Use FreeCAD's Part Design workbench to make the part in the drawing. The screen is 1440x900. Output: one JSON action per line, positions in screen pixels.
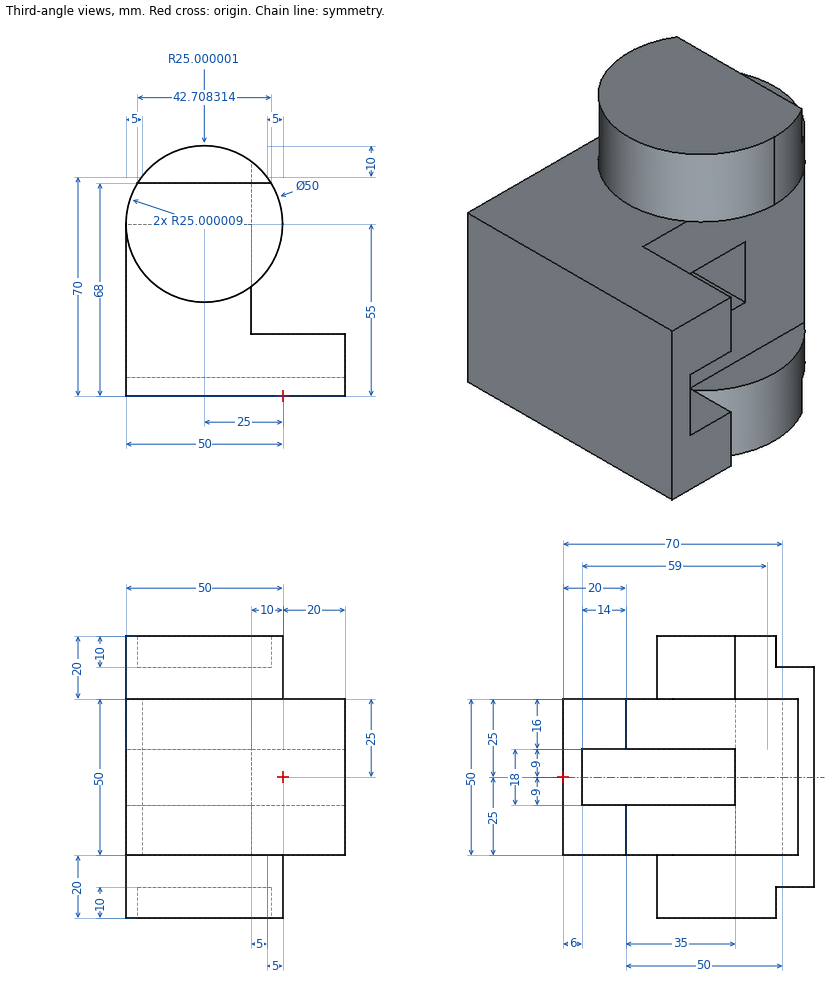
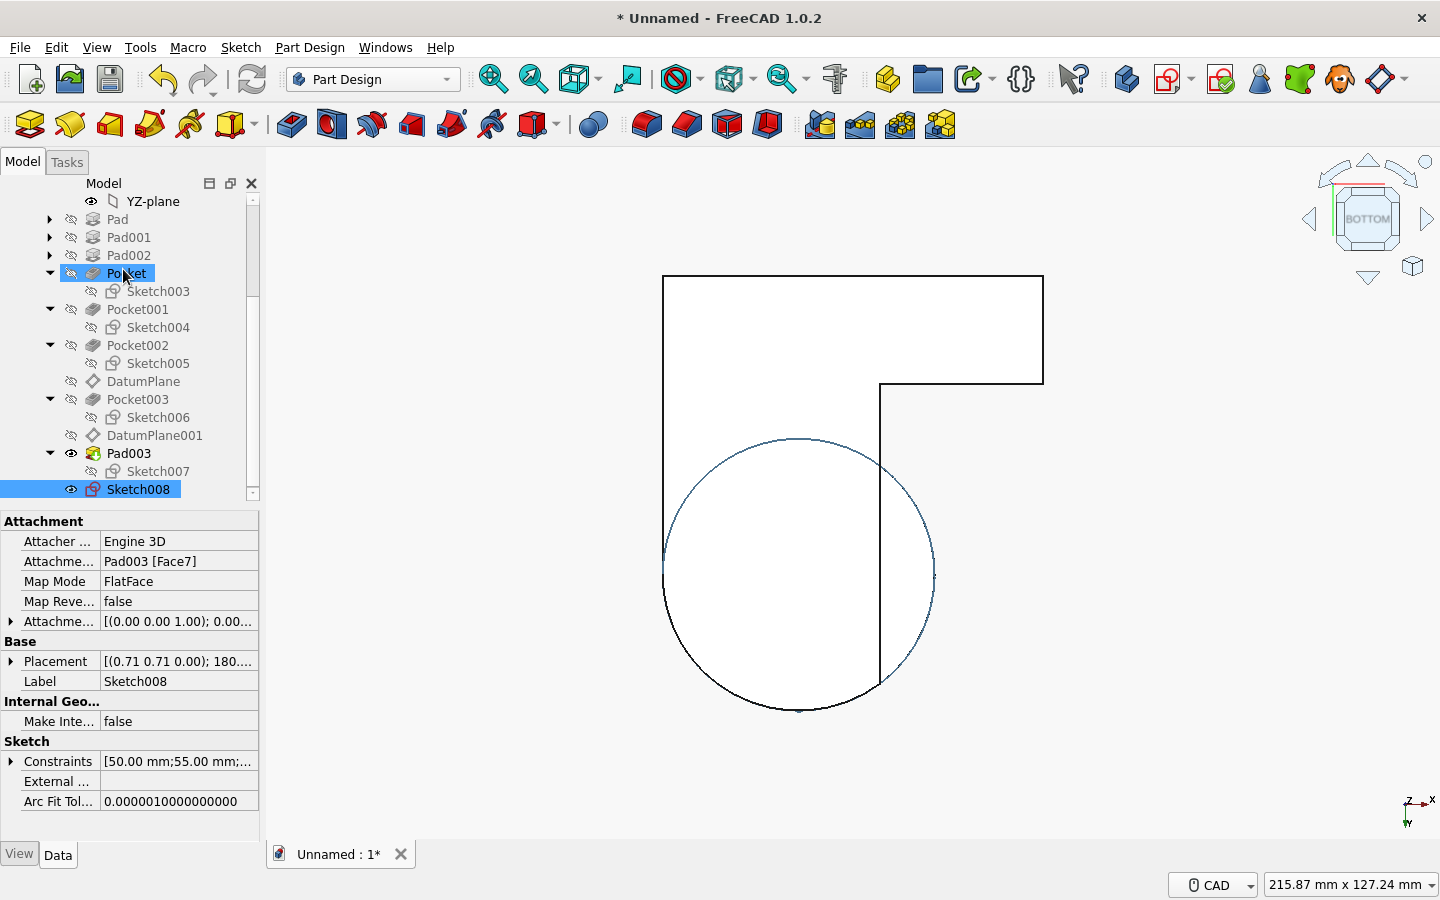
{"action": "left_click", "coordinate": [30, 124]}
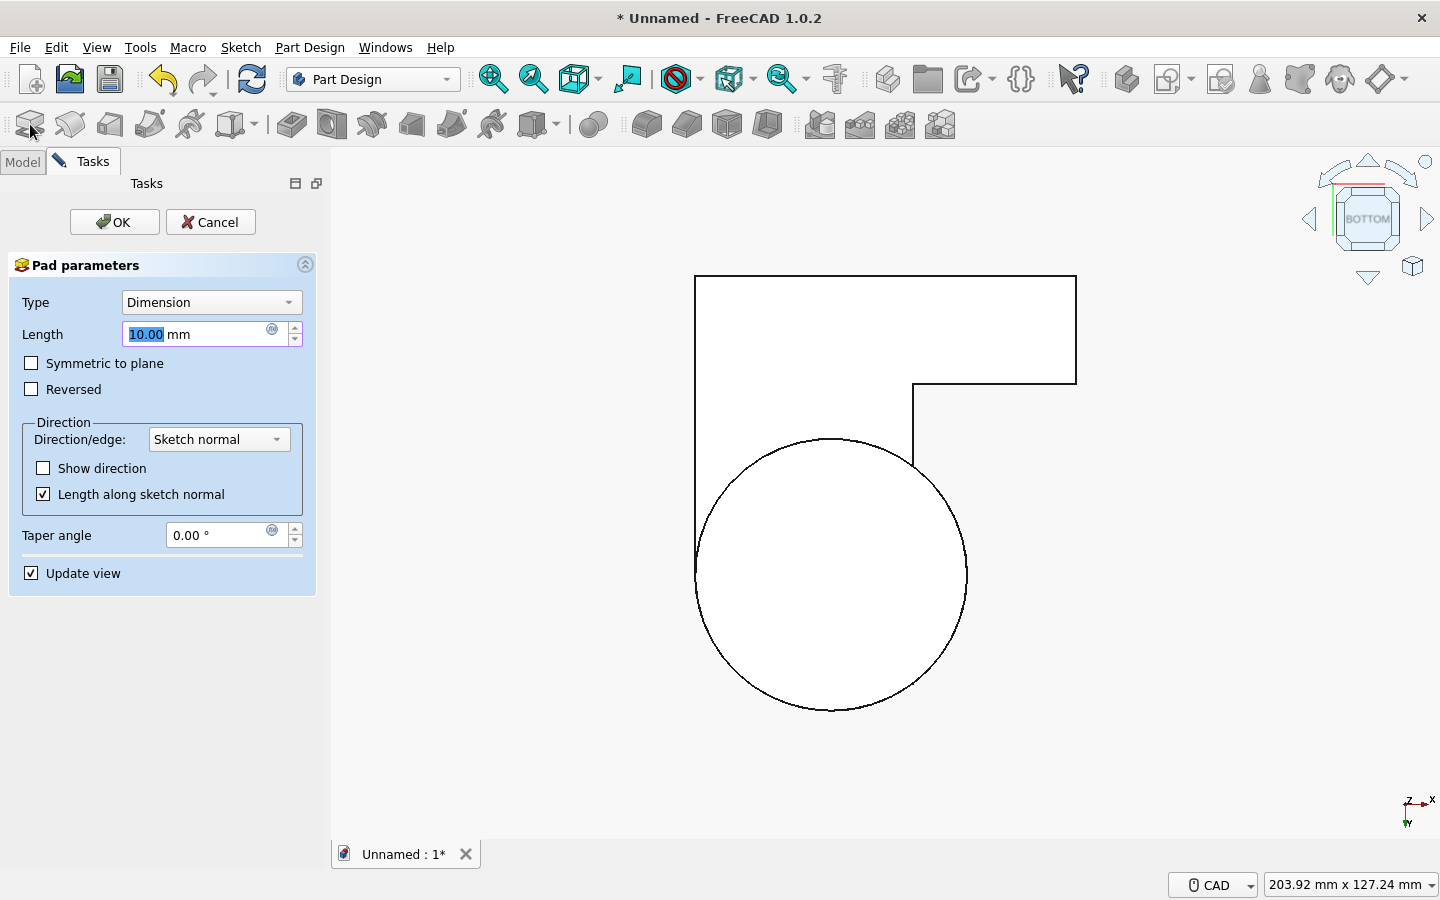
{"action": "type", "text": "20"}
{"action": "key", "text": "Tab"}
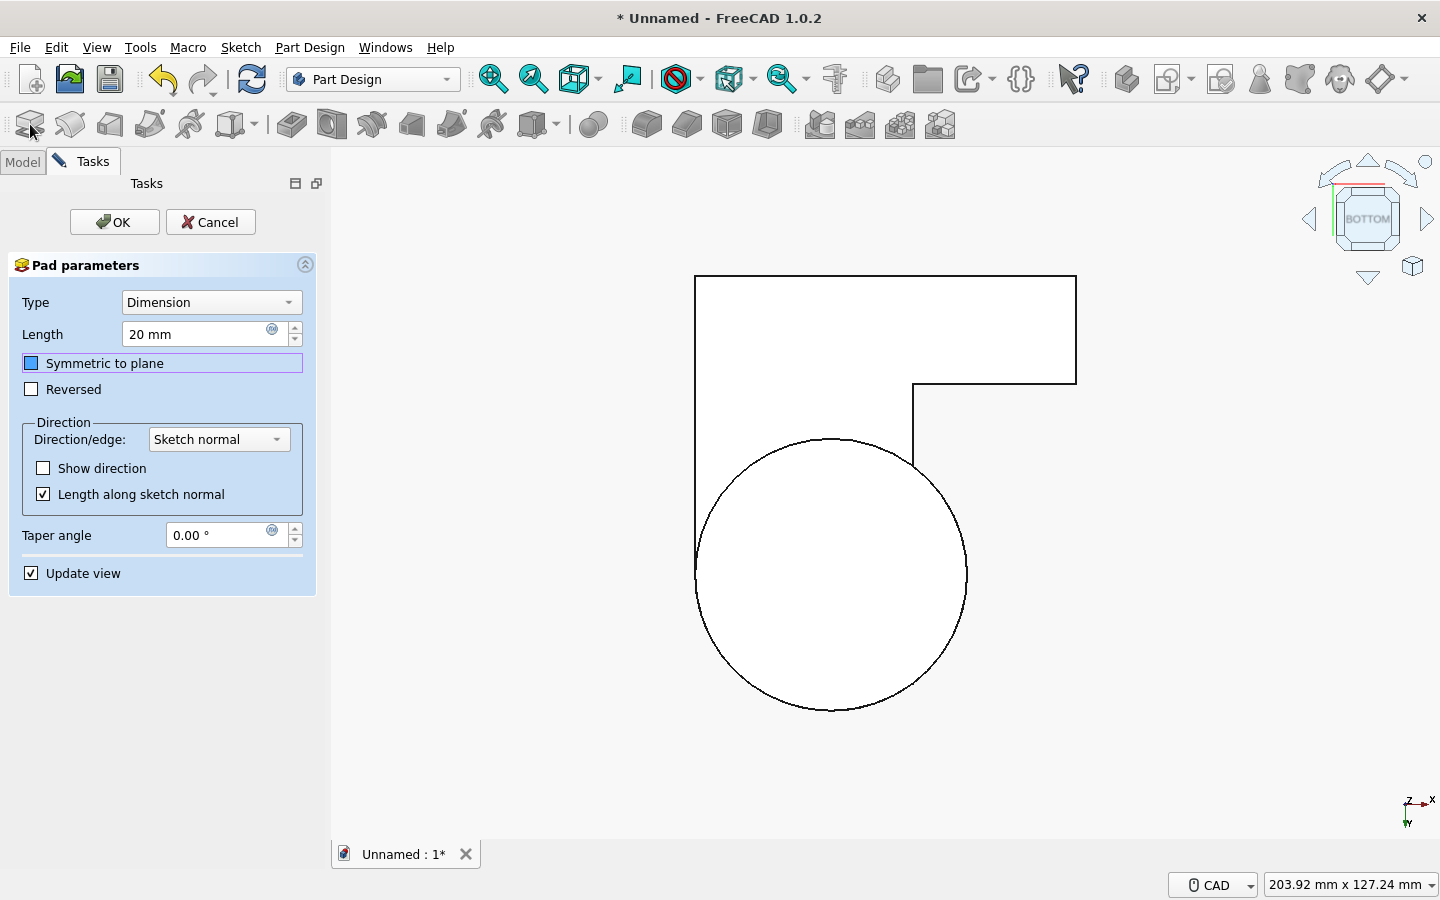
{"action": "left_click", "coordinate": [115, 222]}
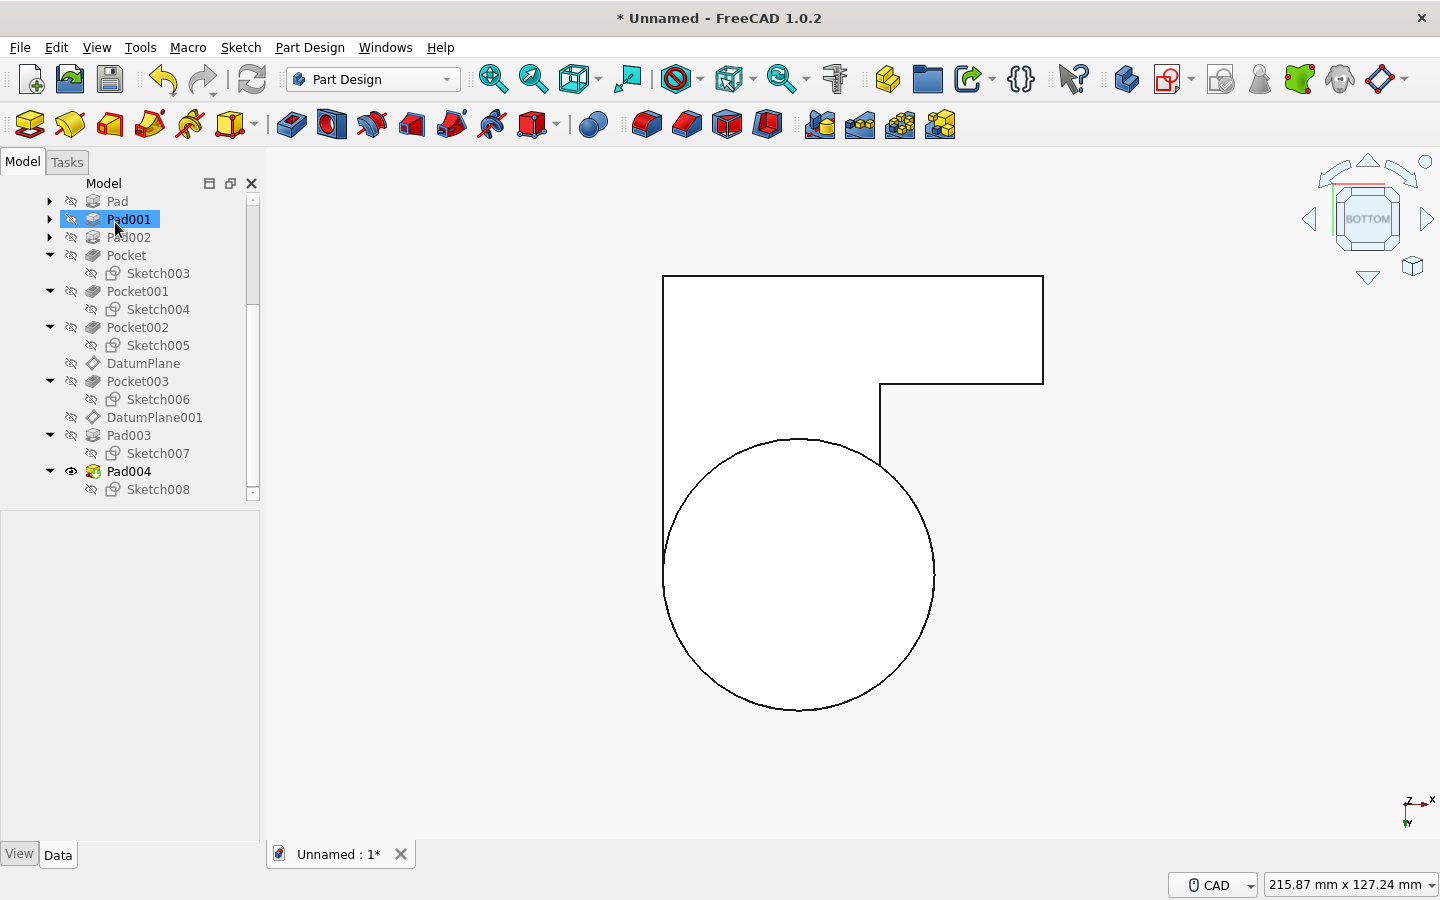
{"action": "key", "text": "0"}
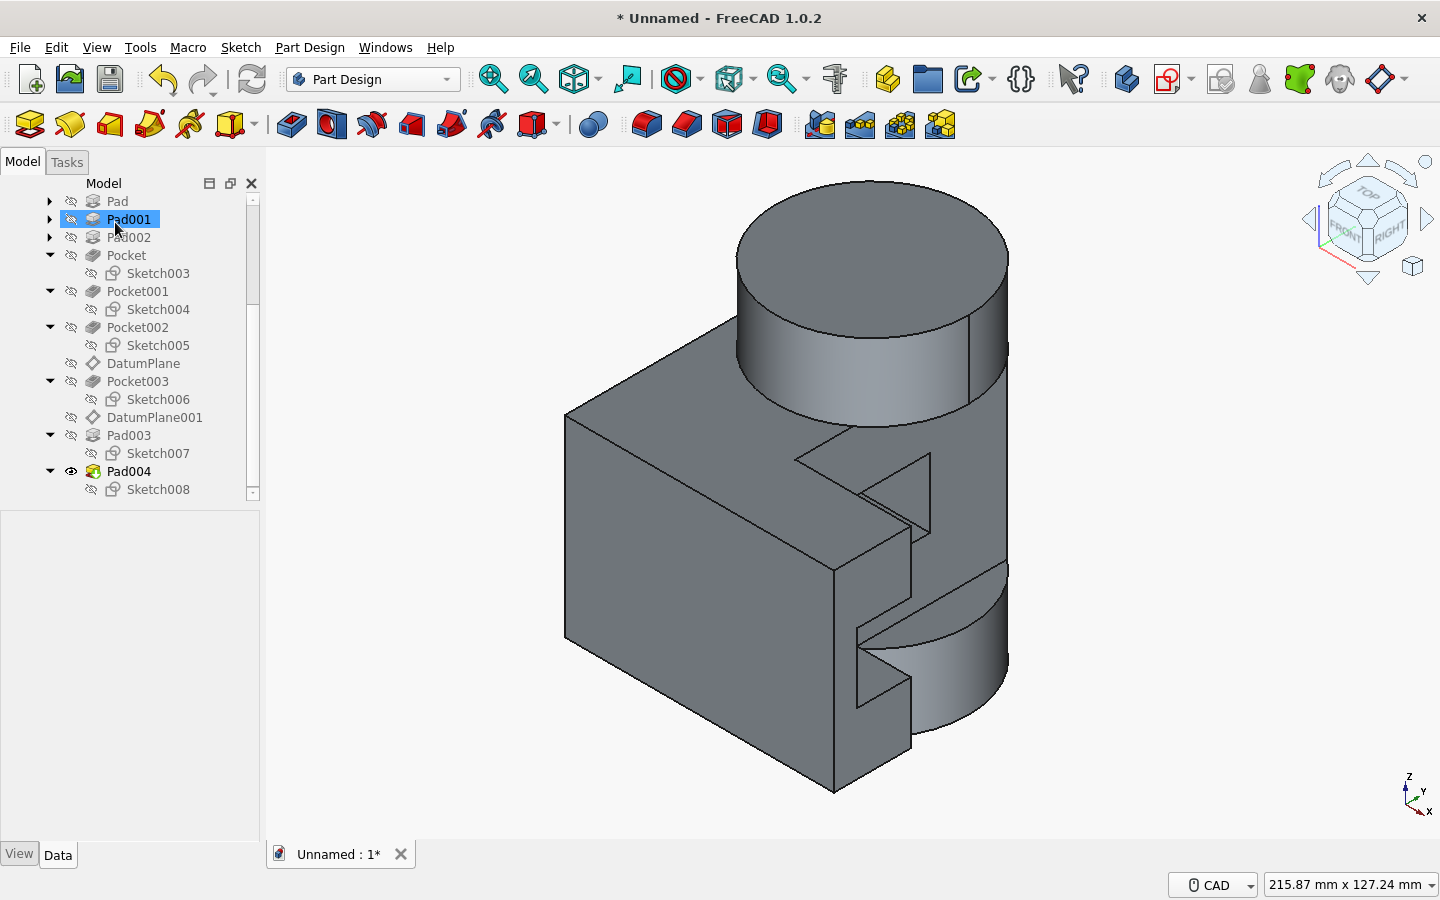
{"action": "left_click", "coordinate": [494, 80]}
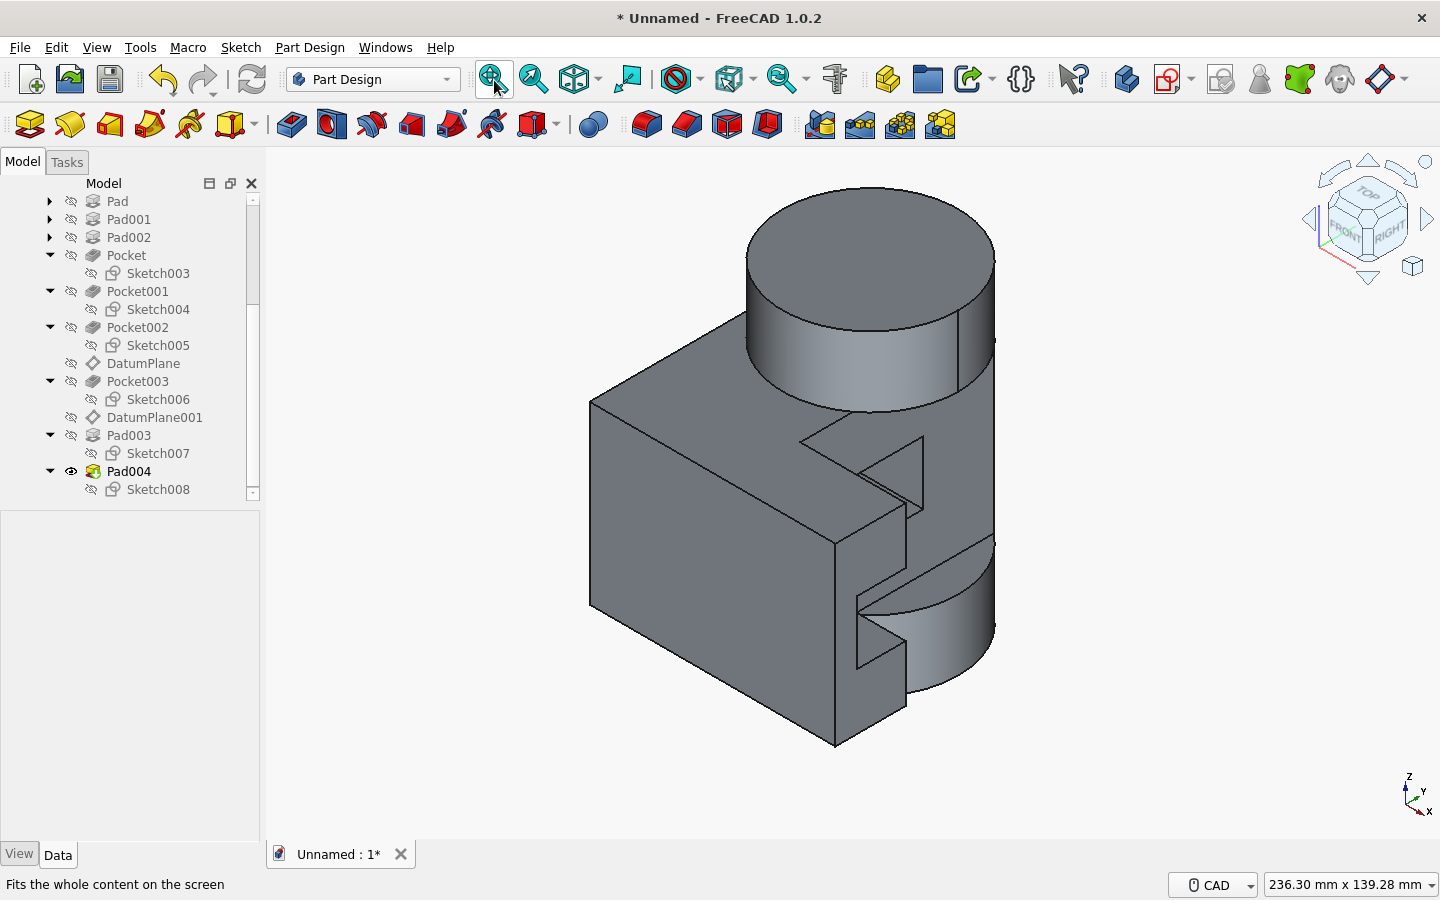
{"action": "left_click", "coordinate": [871, 259]}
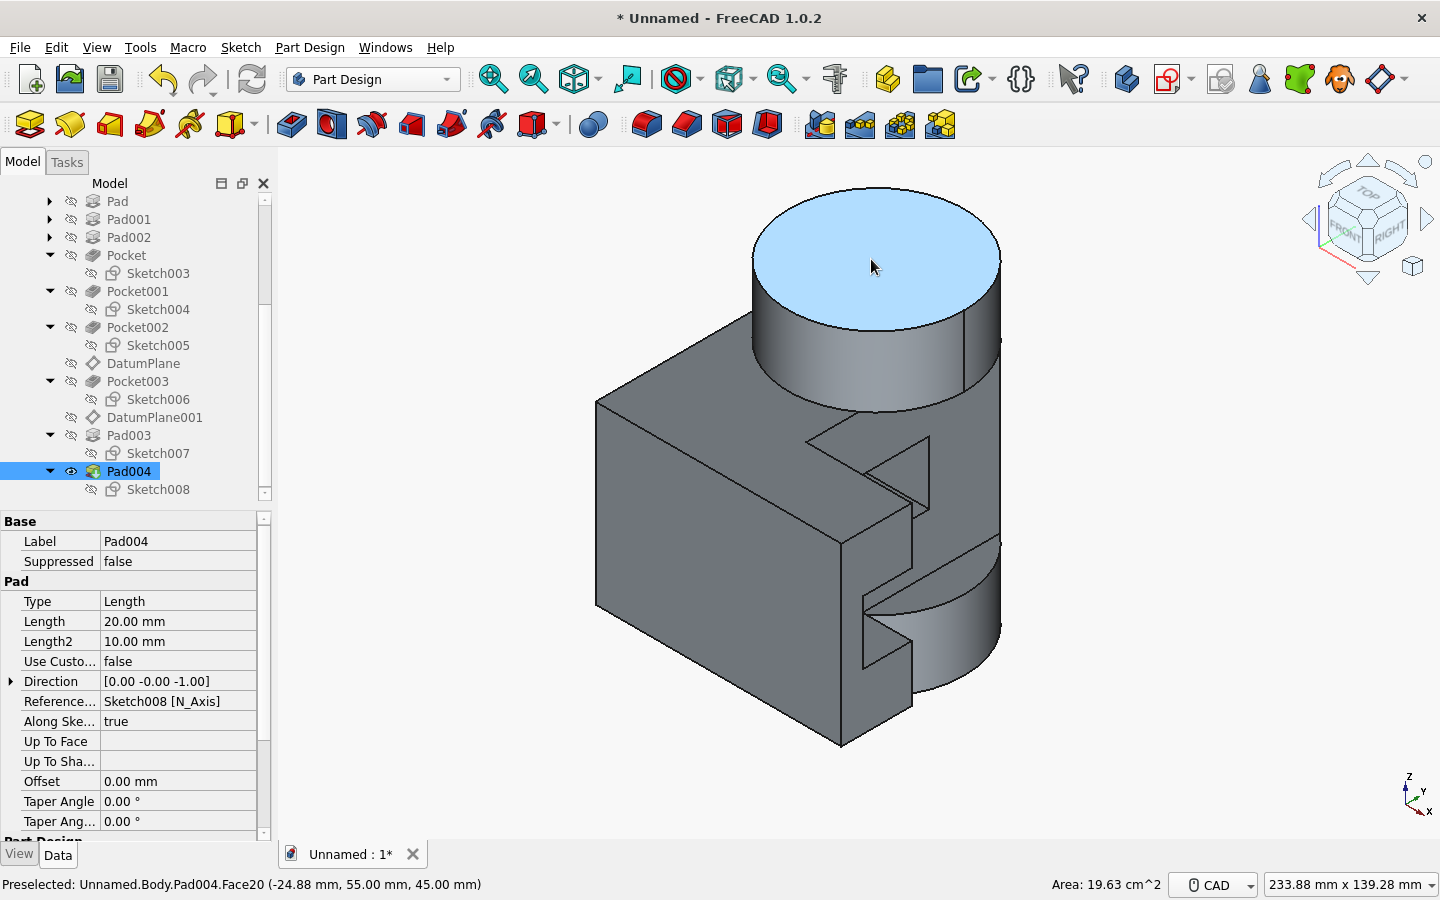
{"action": "left_click", "coordinate": [1168, 80]}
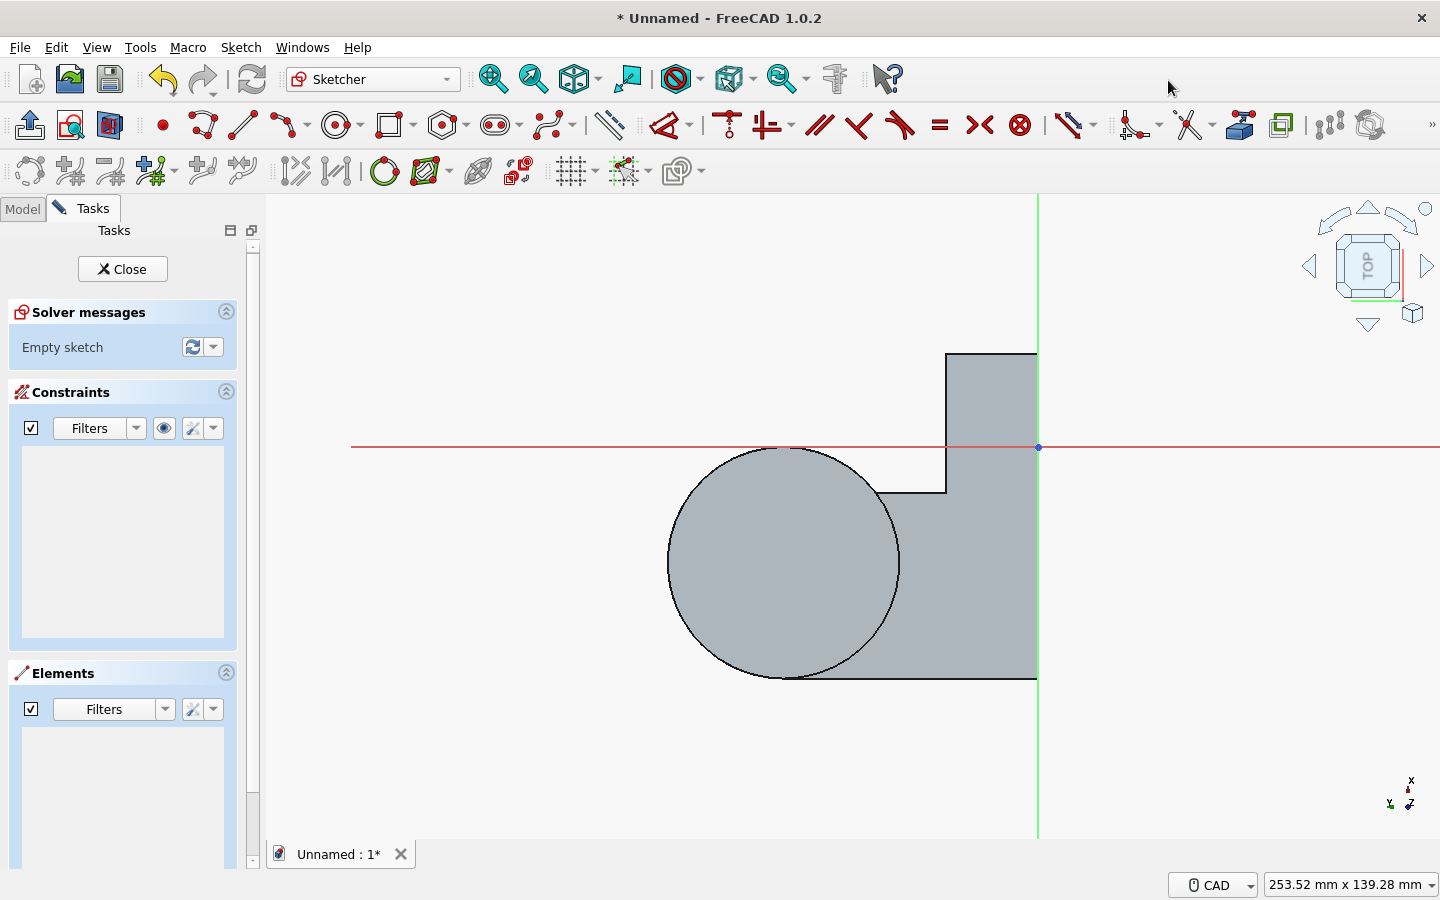
{"action": "scroll", "coordinate": [936, 600], "scroll_direction": "up", "scroll_amount": 3}